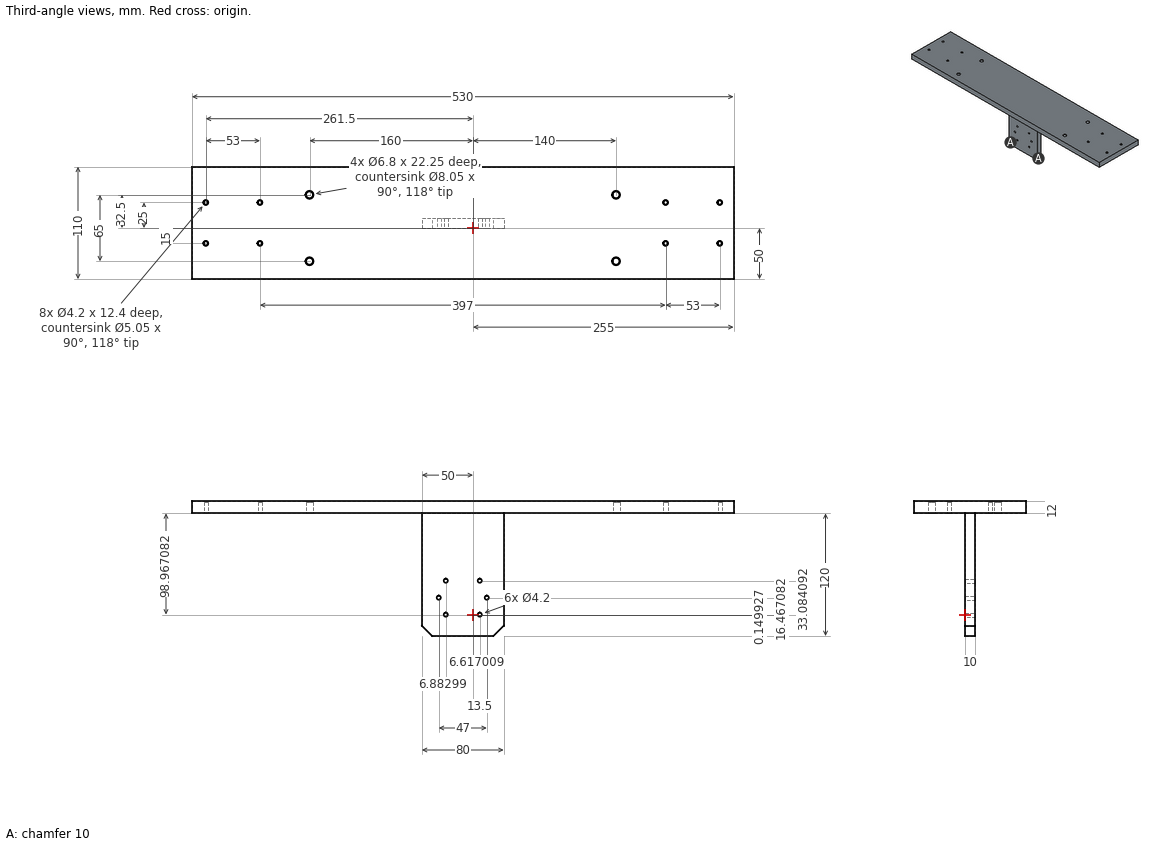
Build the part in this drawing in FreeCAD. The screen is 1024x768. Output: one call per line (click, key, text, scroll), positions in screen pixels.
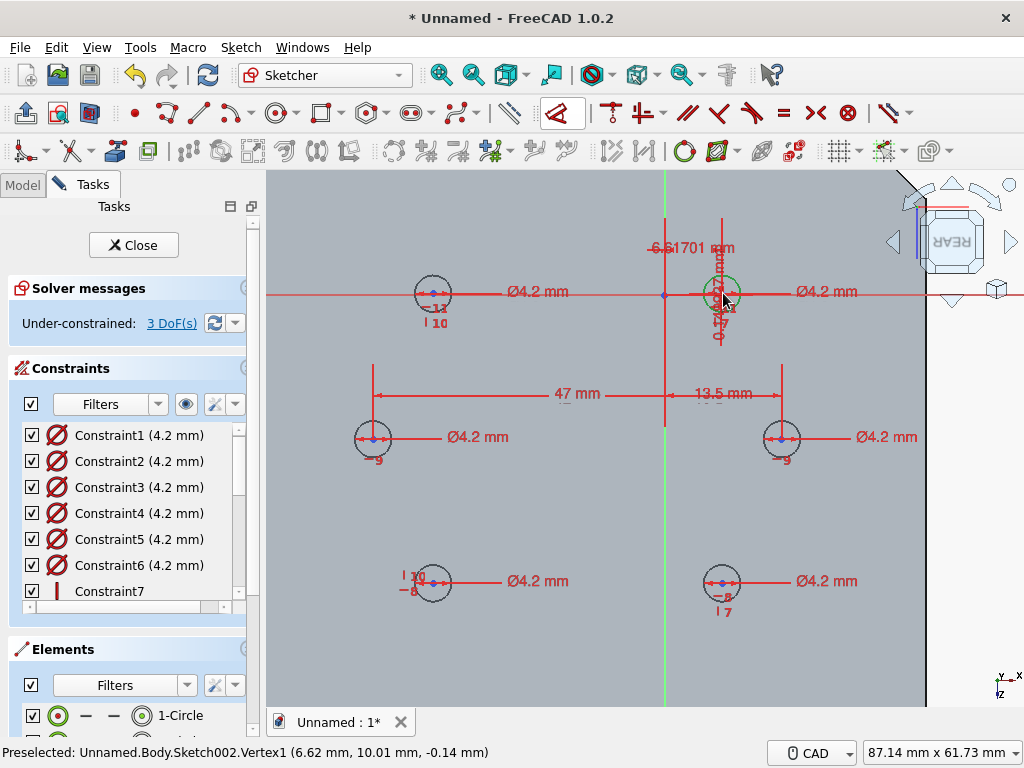
click(433, 583)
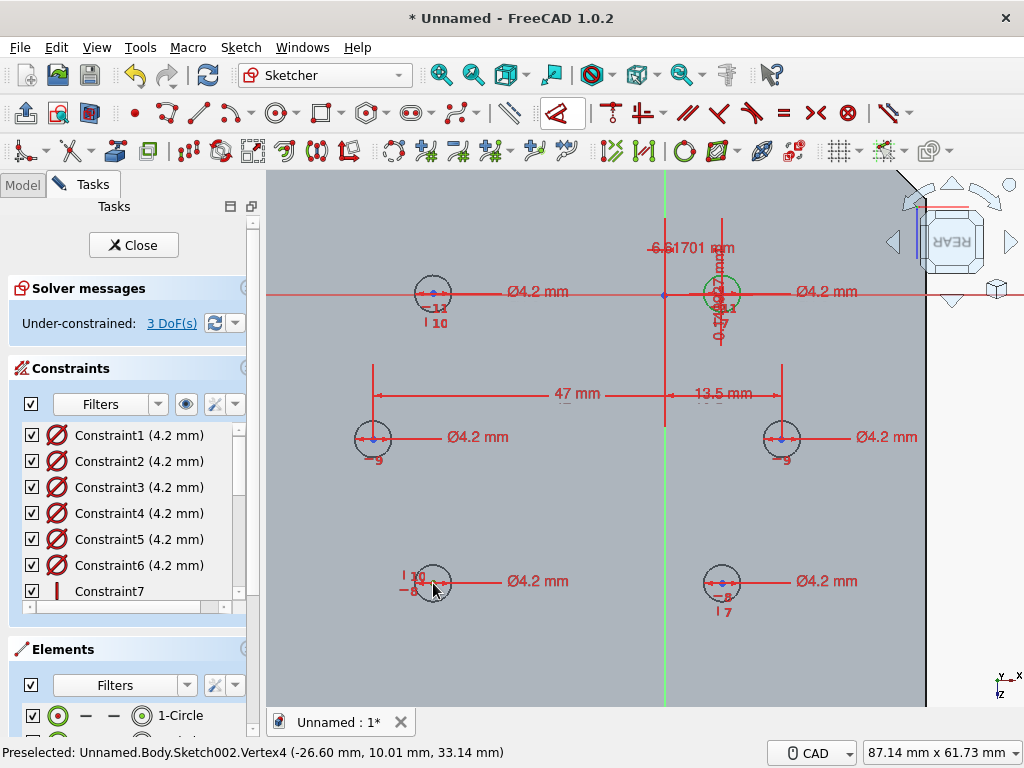
click(373, 439)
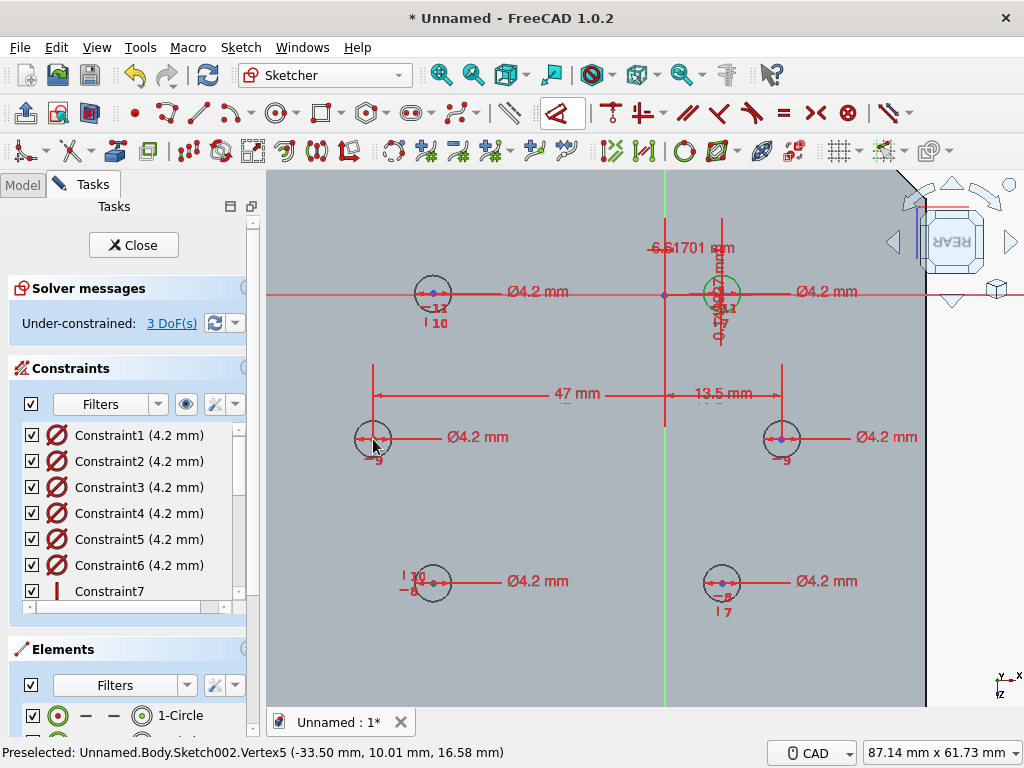
key(l)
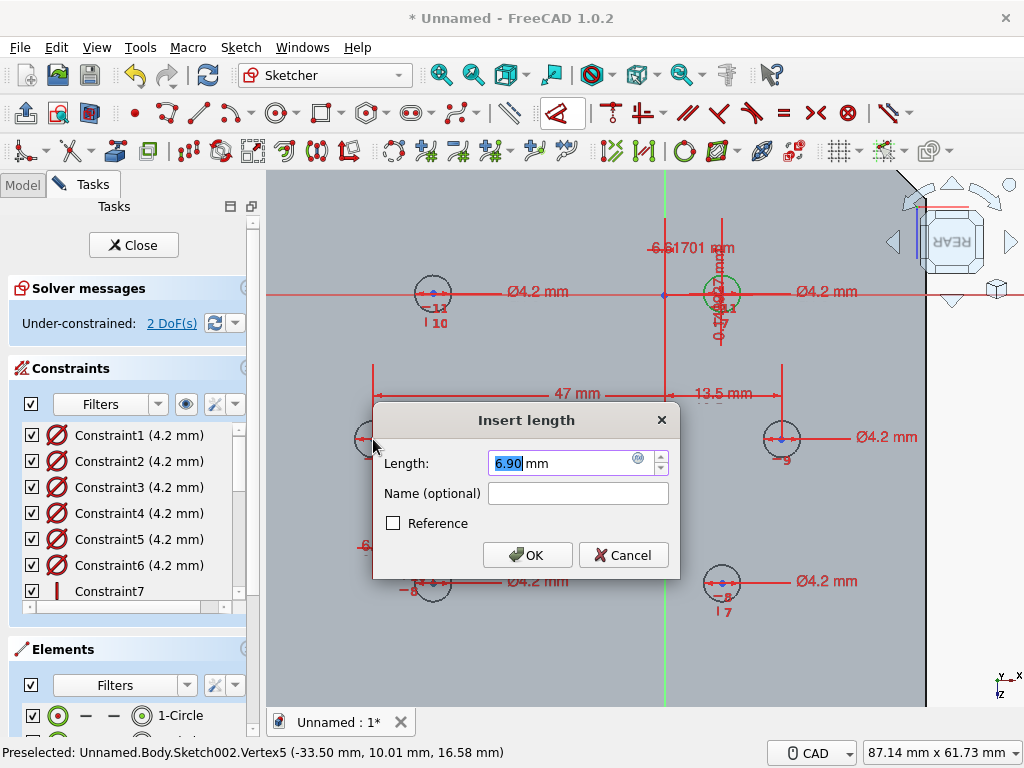
text(6.88299)
key(Return)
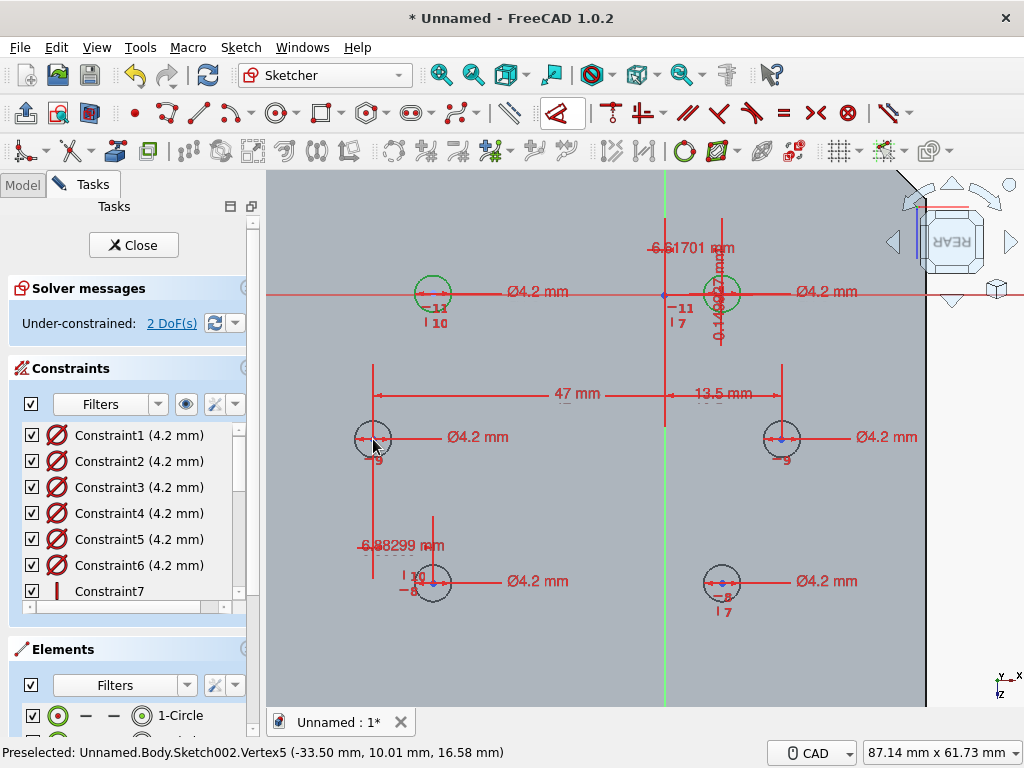
click(782, 439)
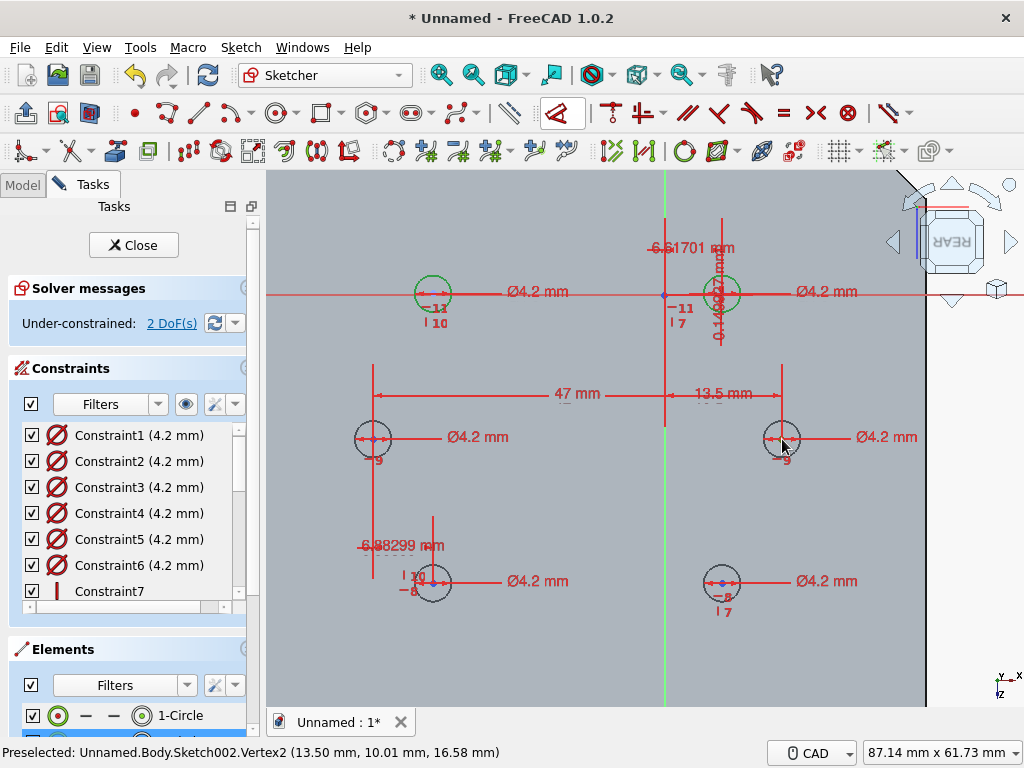
key(i)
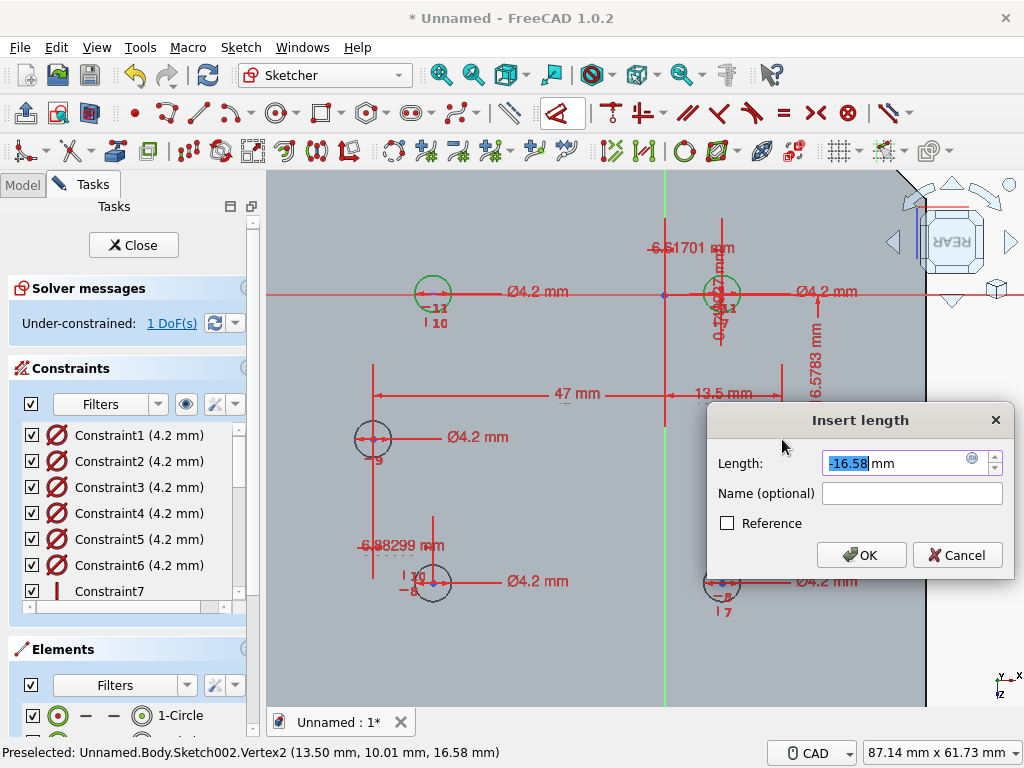
text(-16.467082)
key(Return)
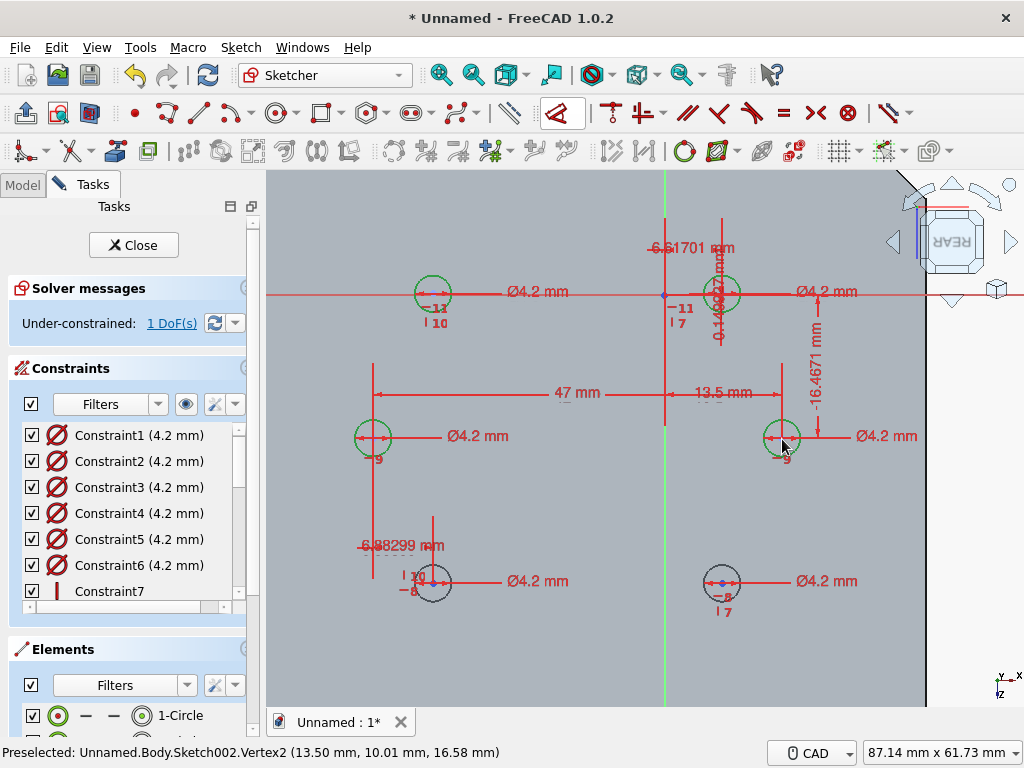
click(722, 583)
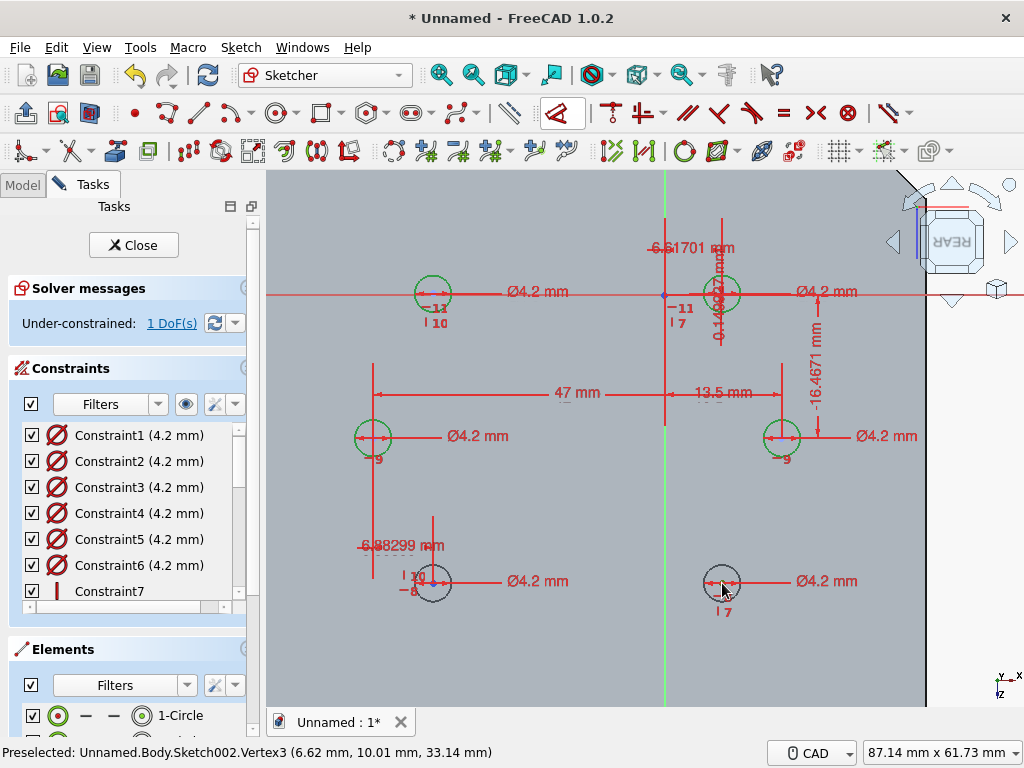
click(580, 114)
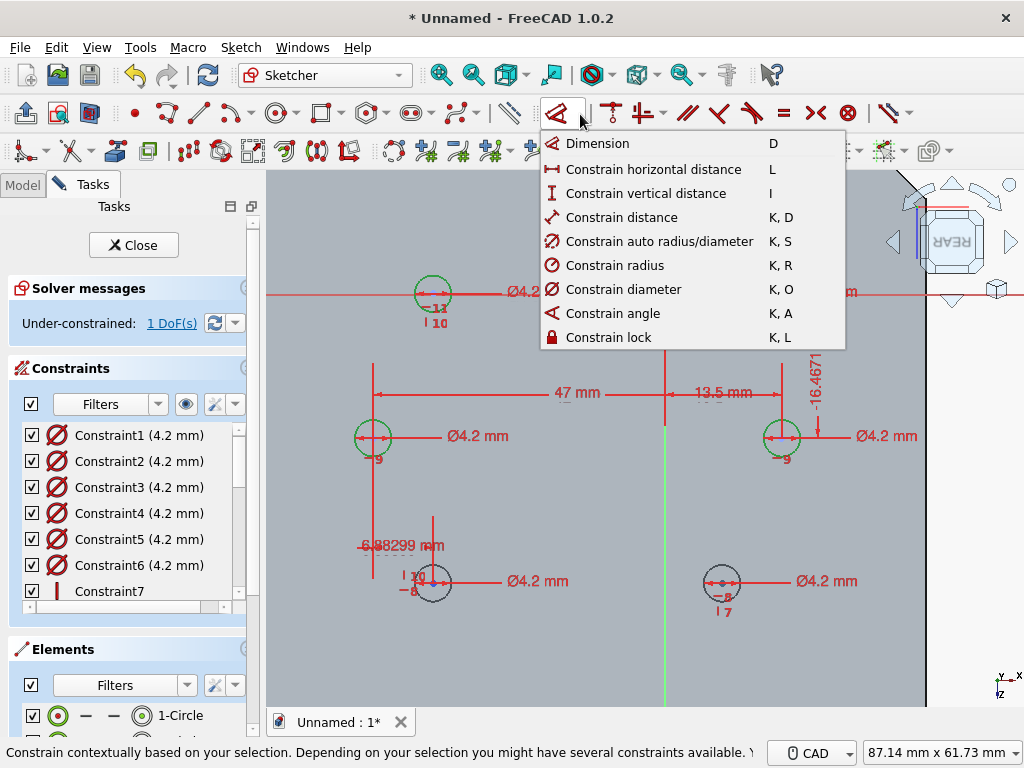
click(693, 193)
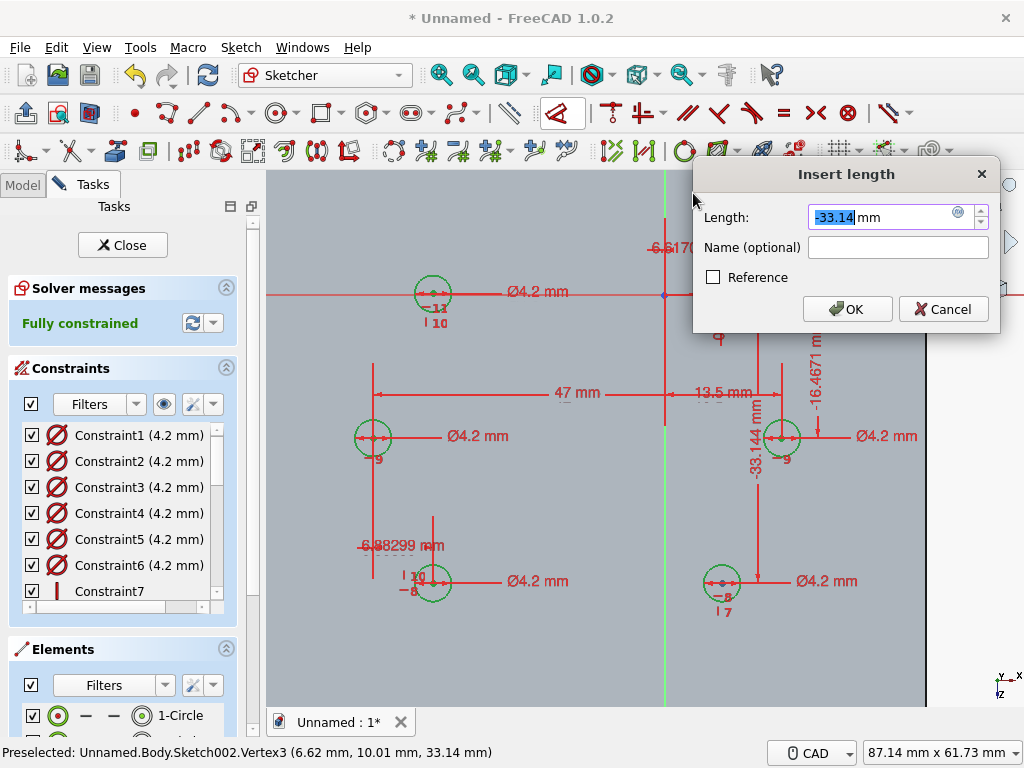
text(-33.084092)
key(Return)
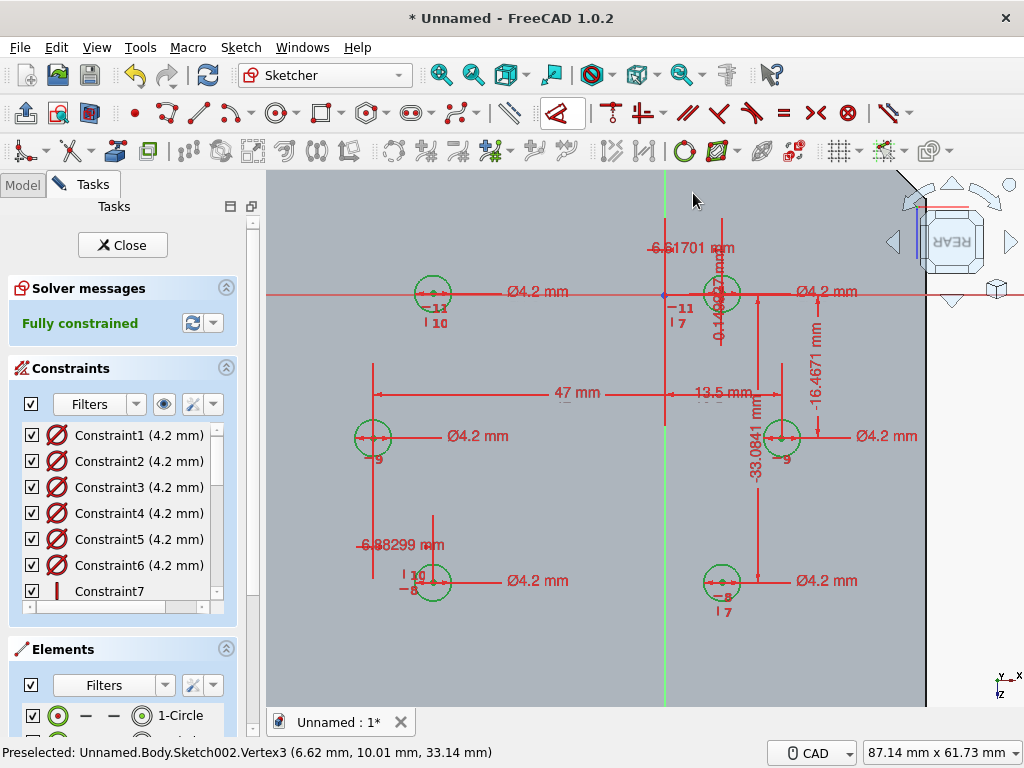
click(123, 245)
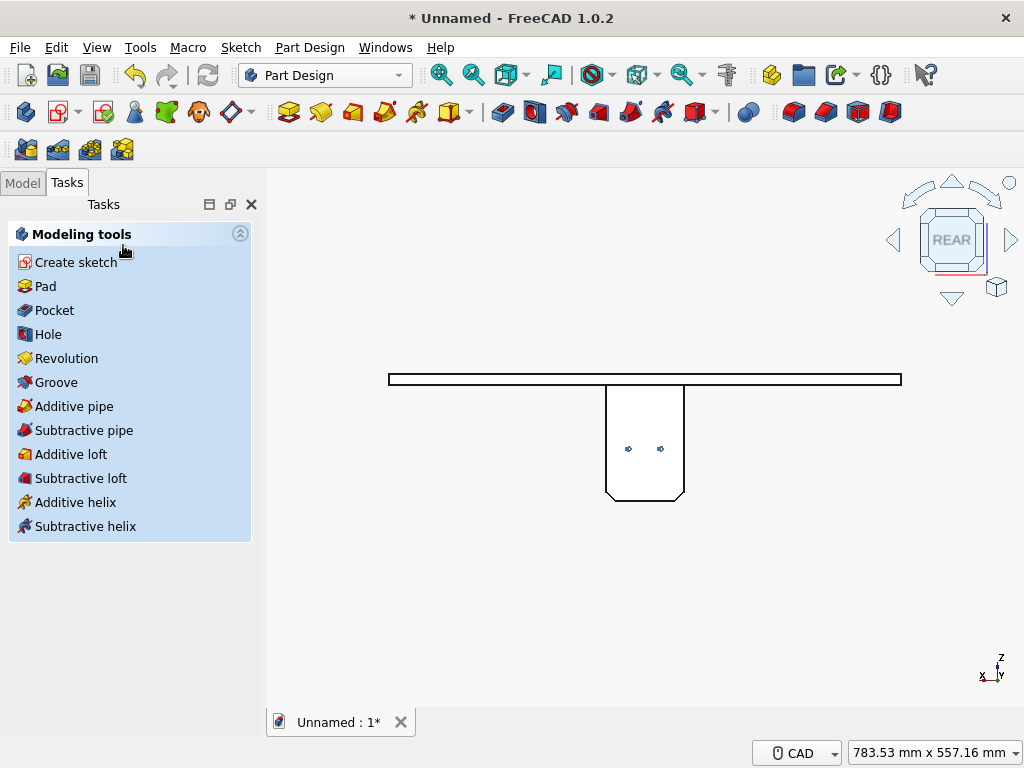
click(504, 112)